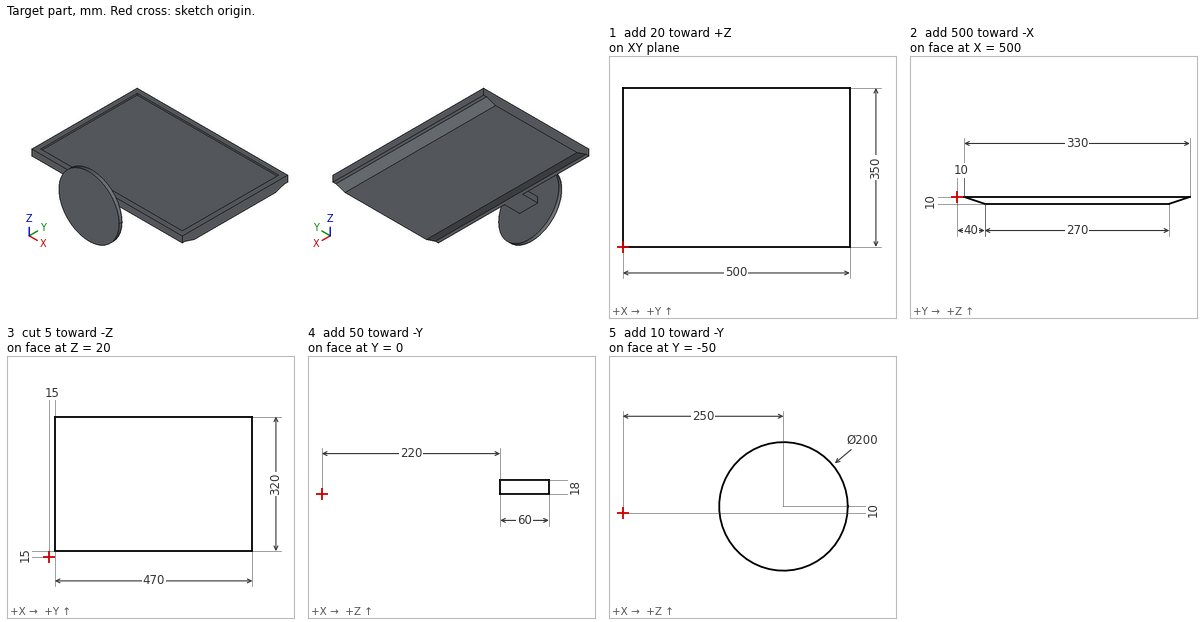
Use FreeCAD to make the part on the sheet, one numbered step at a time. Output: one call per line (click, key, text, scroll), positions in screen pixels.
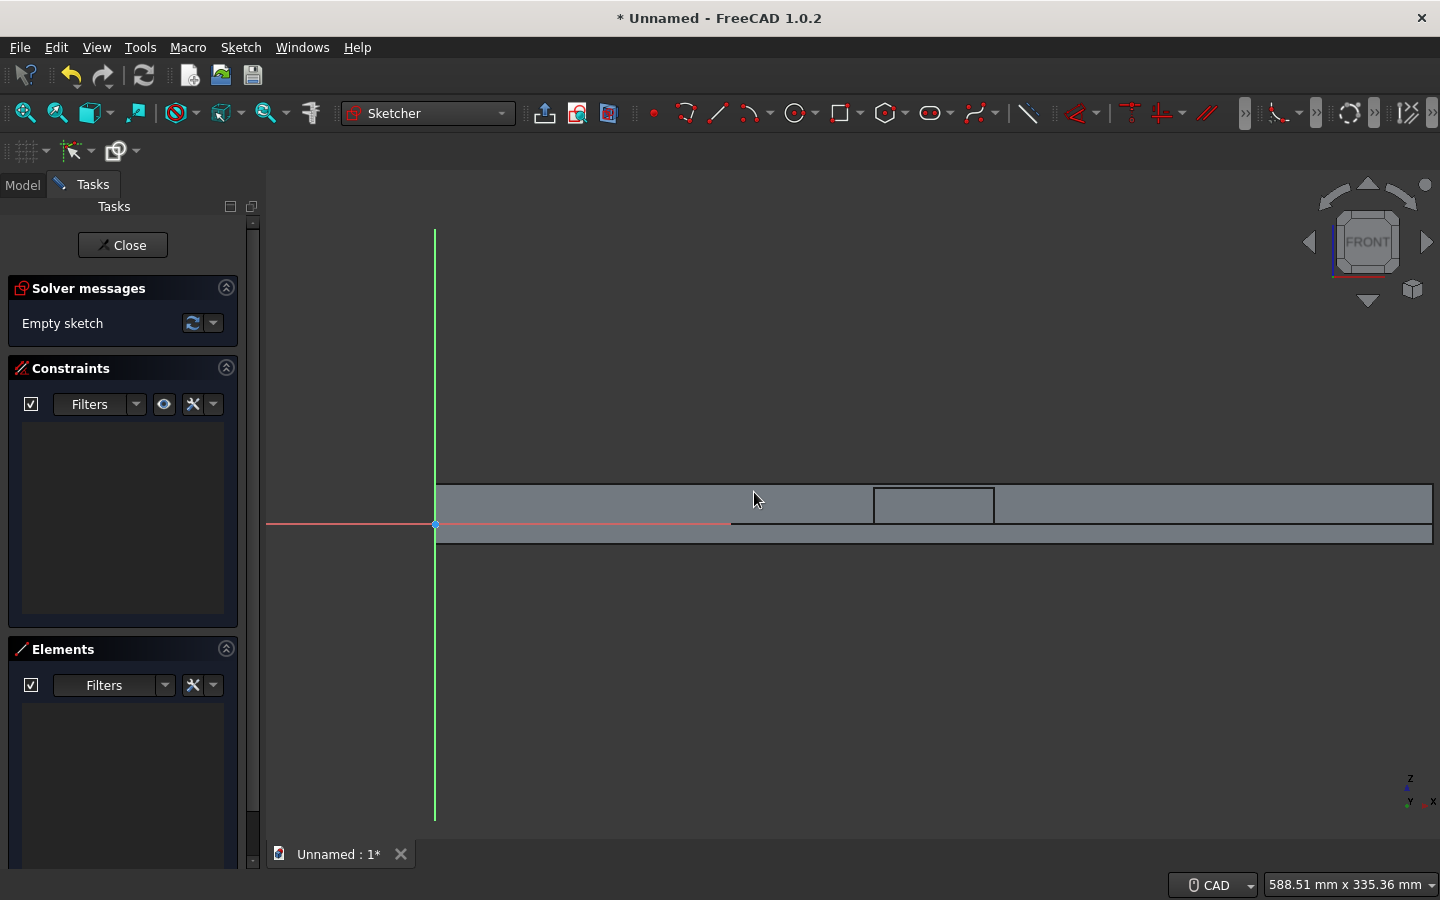
key(g)
key(c)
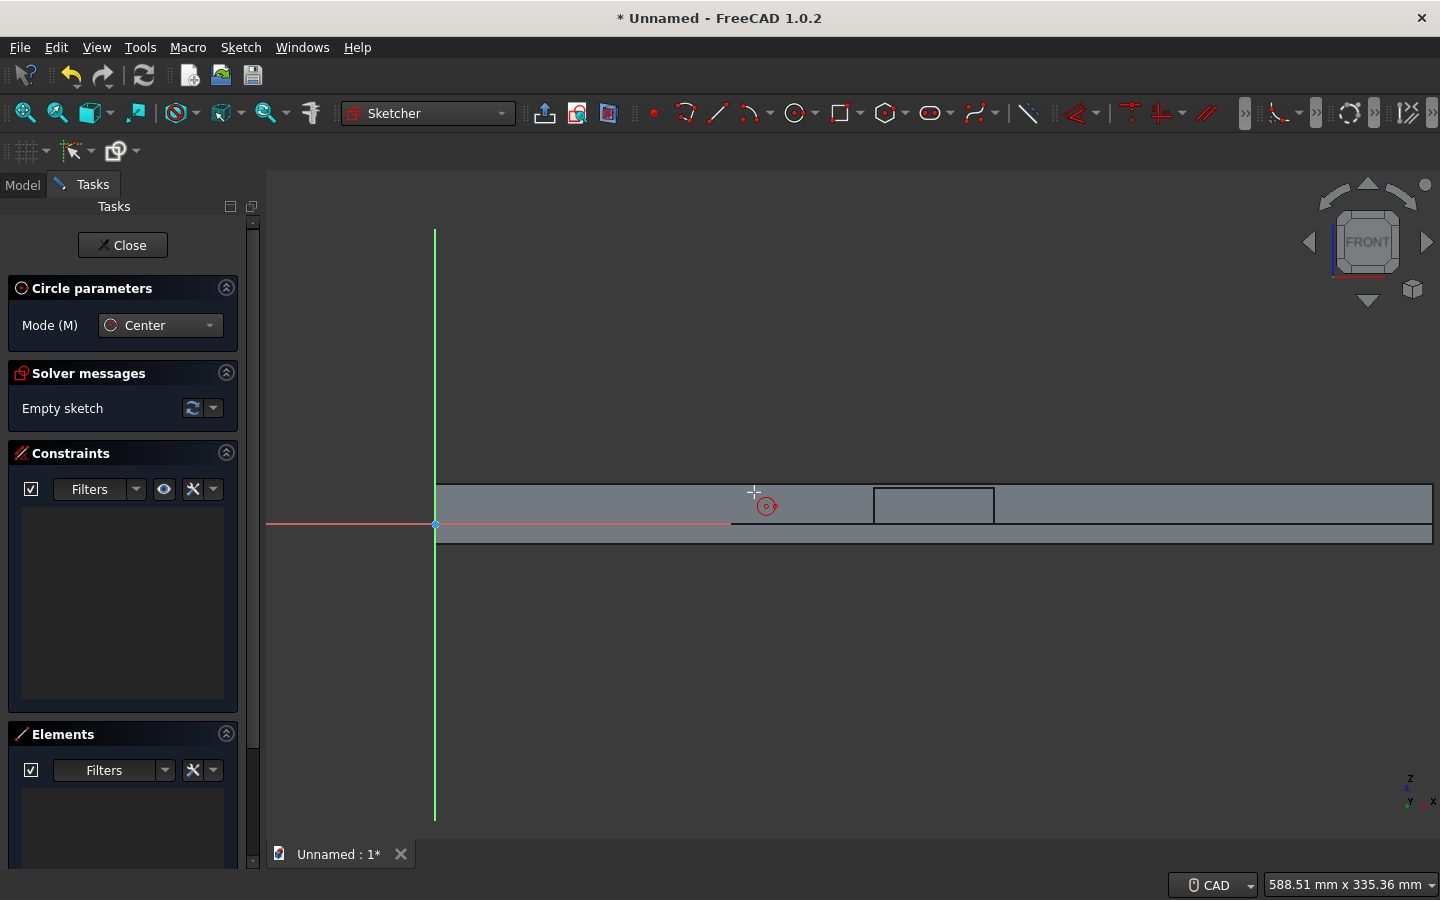
click(934, 504)
move(1075, 363)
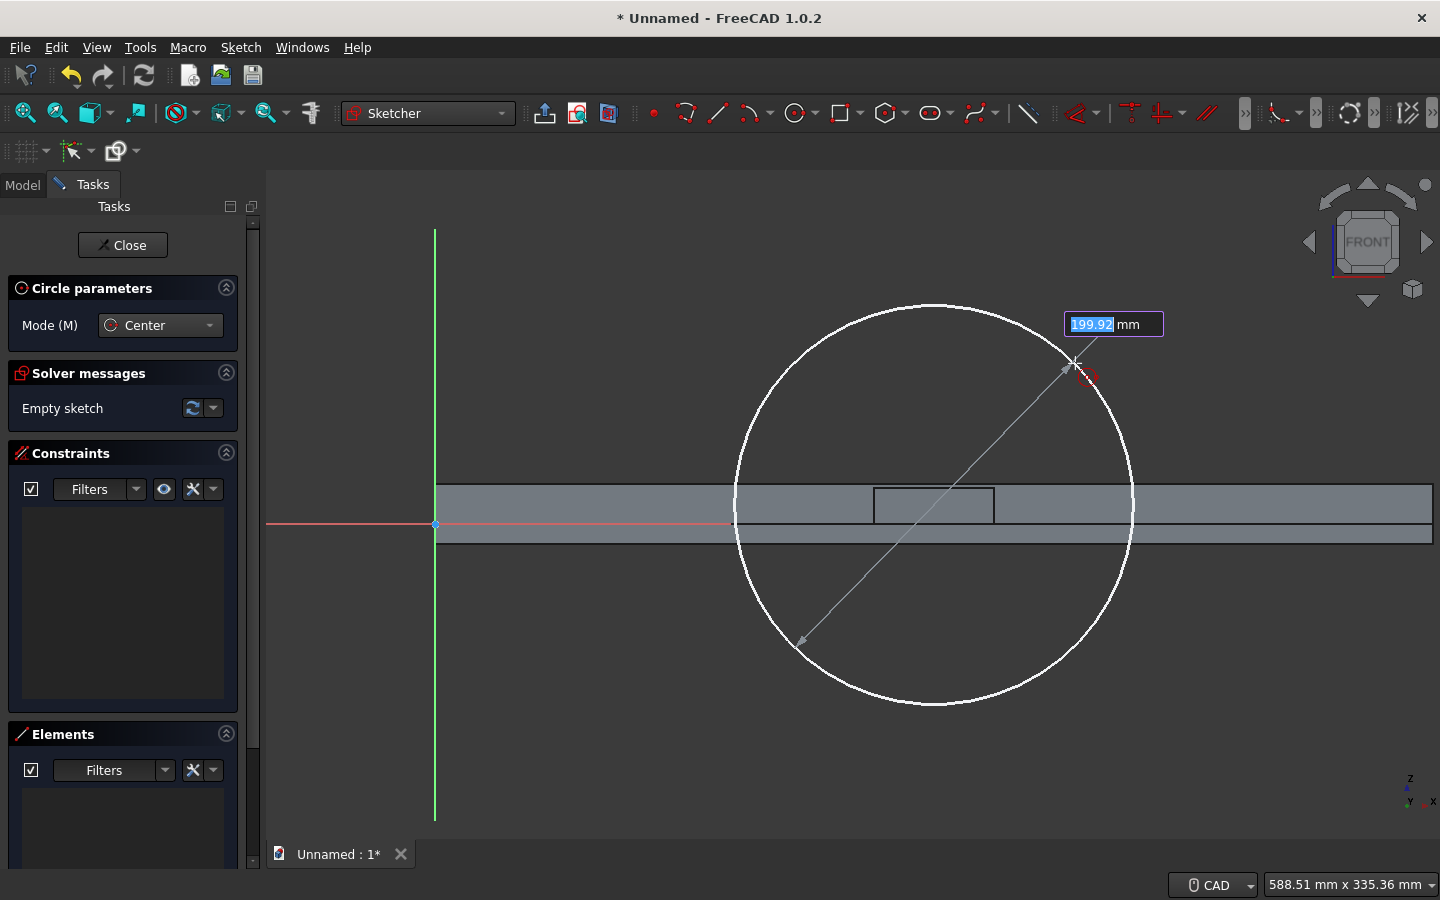
text(200)
key(Return)
key(Escape)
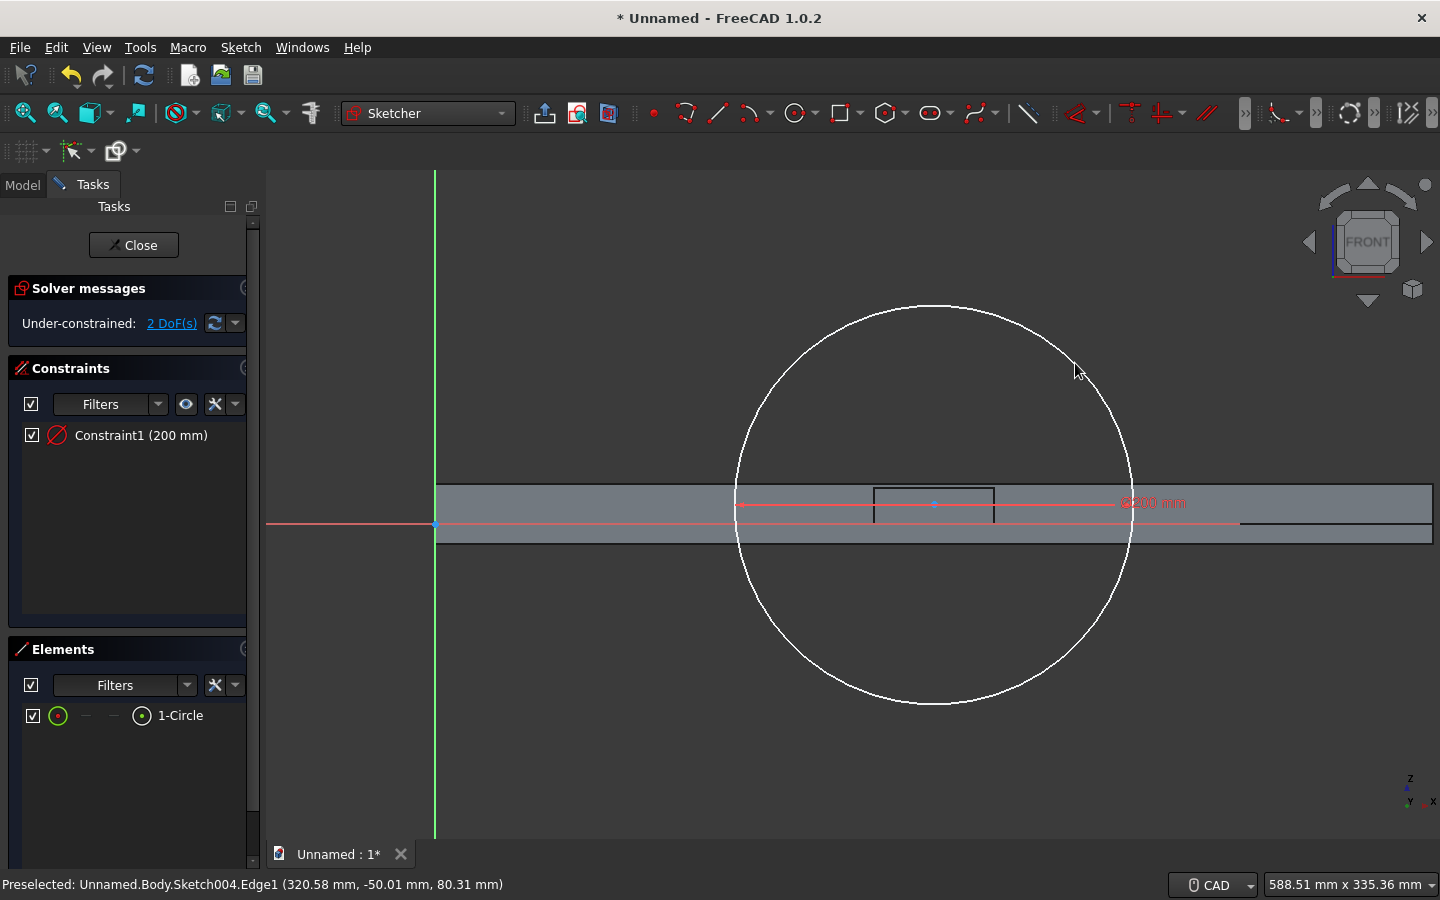
key(d)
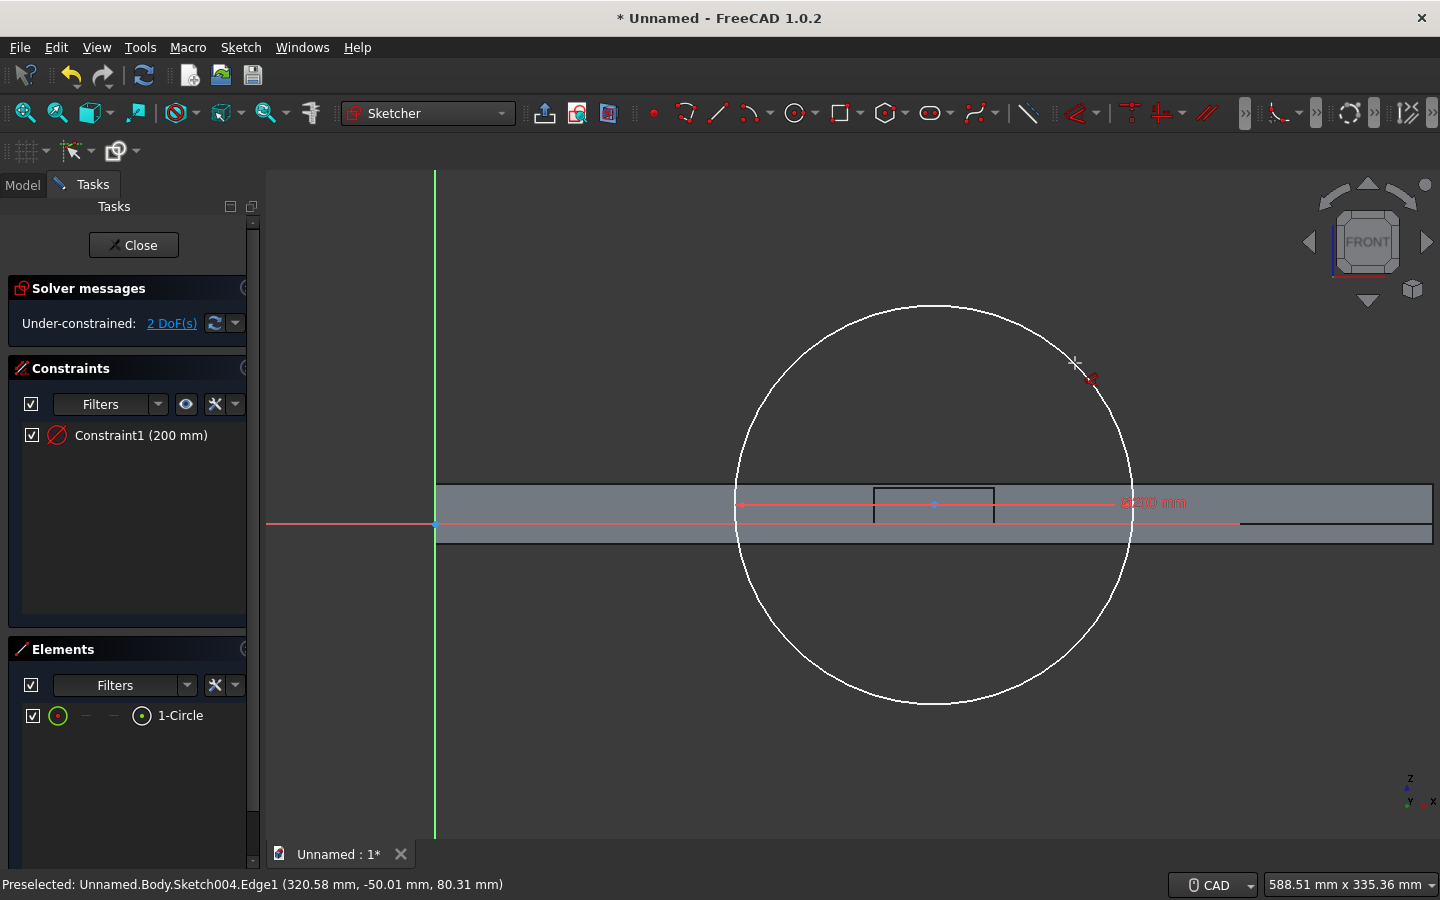
scroll(934, 505, up, 4)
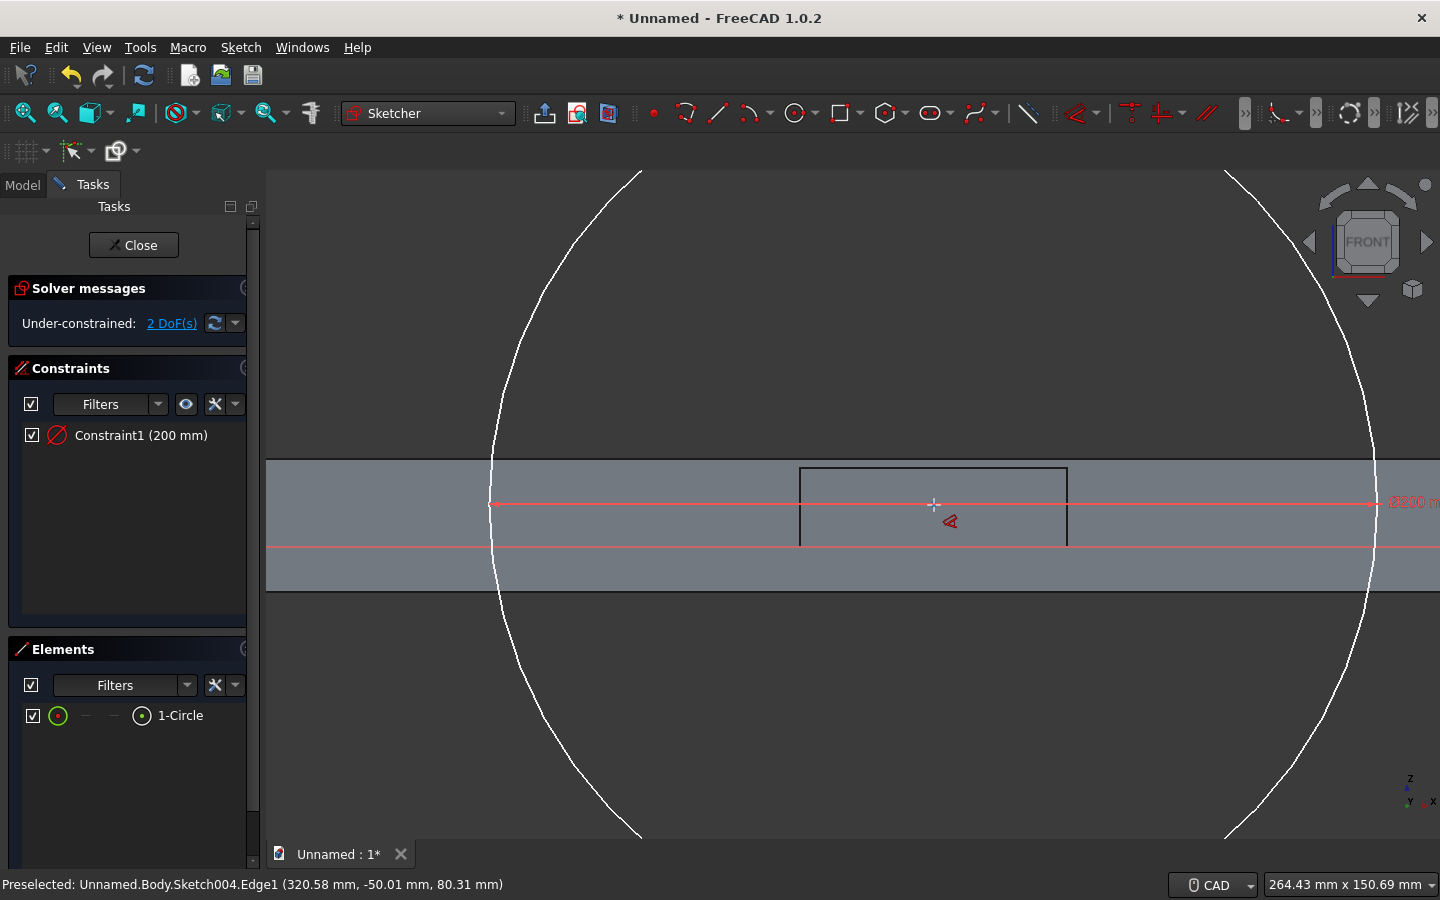
click(933, 504)
click(967, 526)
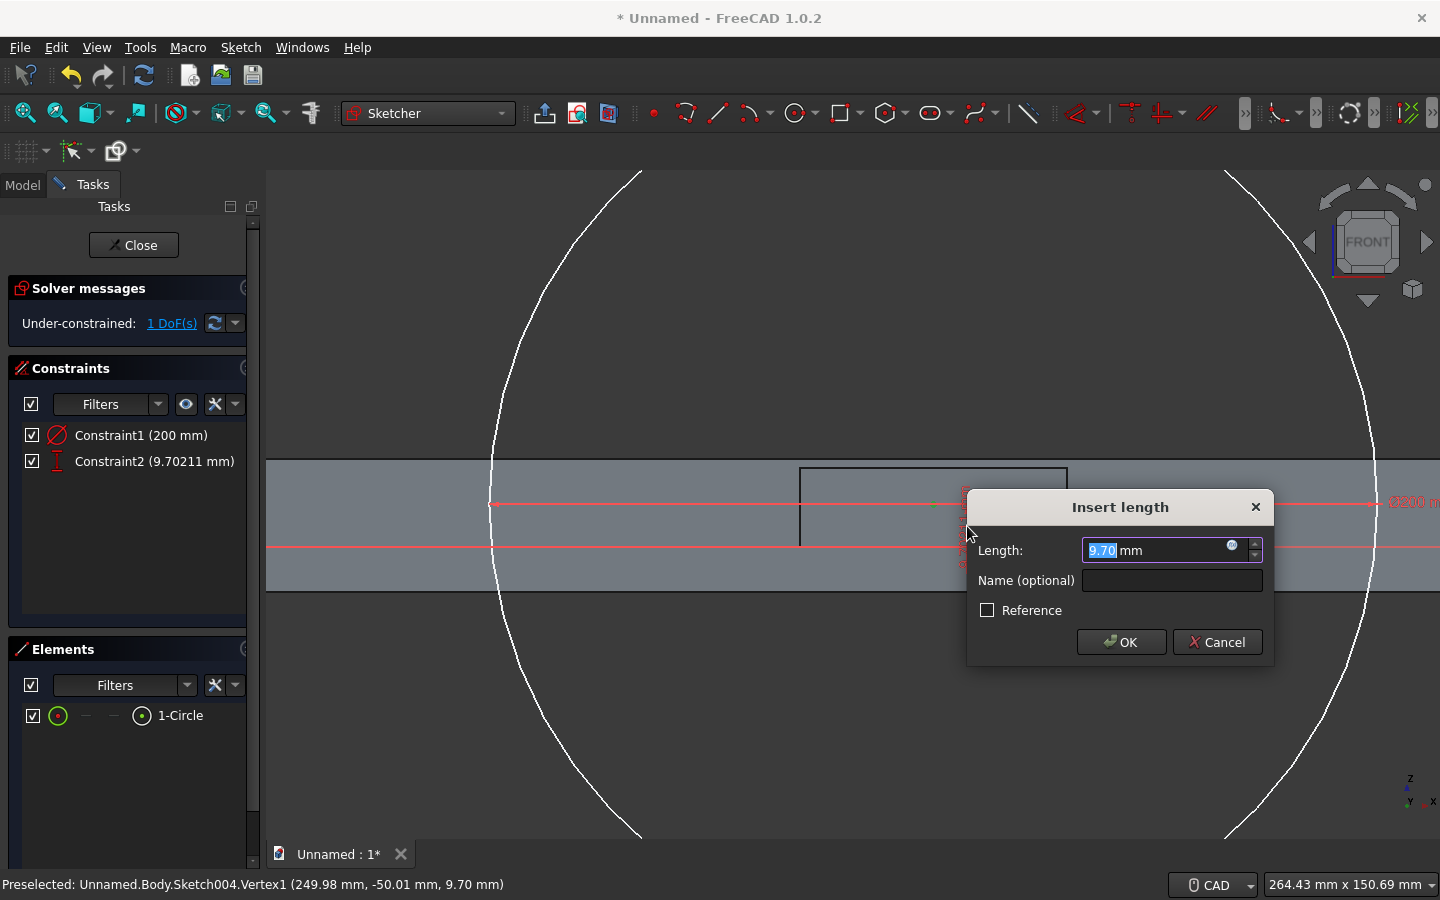
text(10)
key(Return)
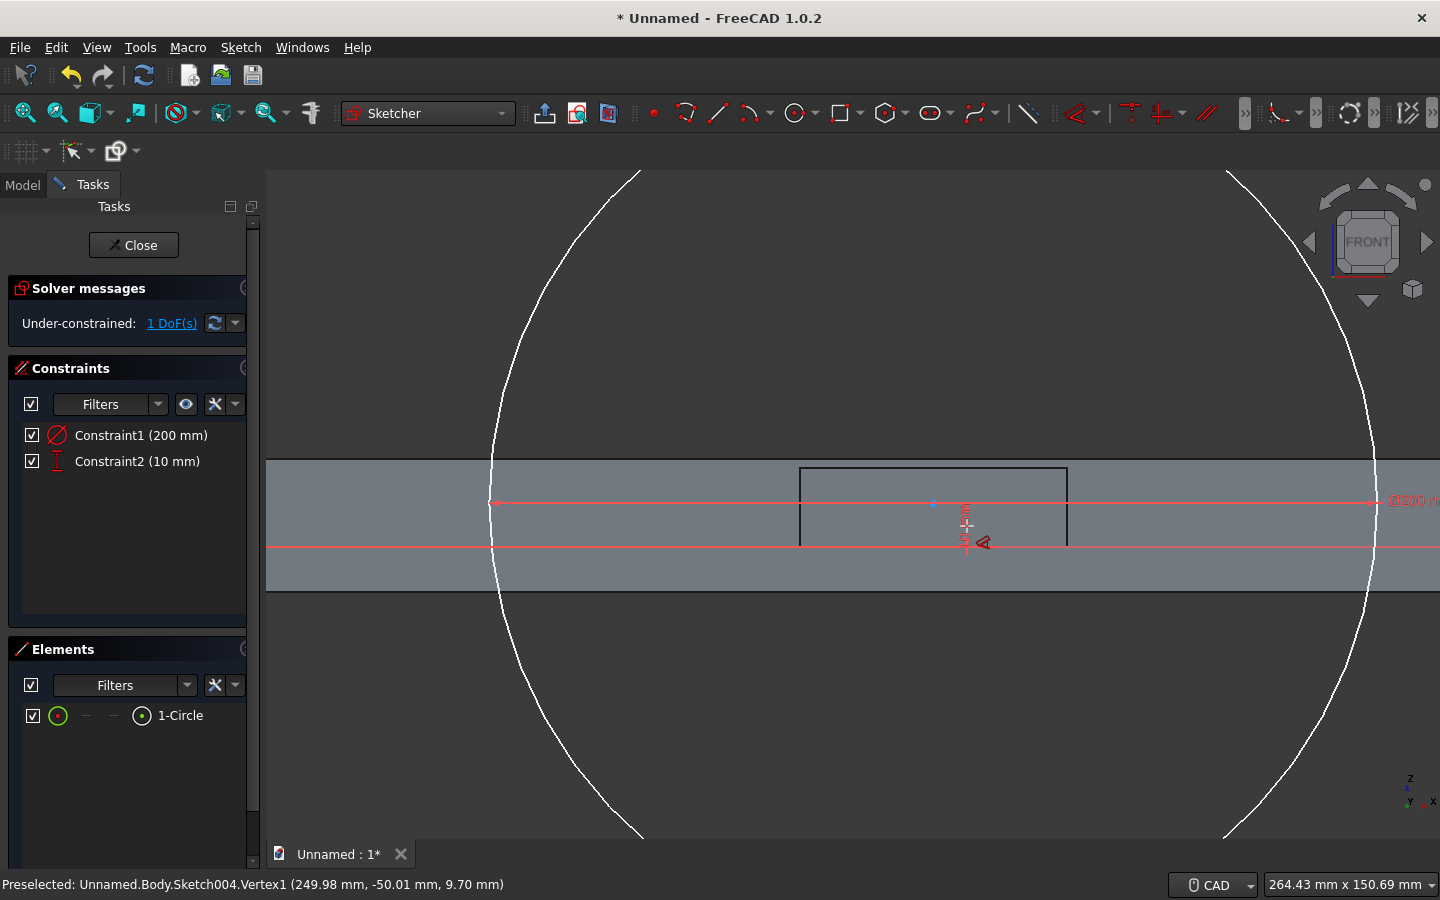
click(933, 503)
click(614, 581)